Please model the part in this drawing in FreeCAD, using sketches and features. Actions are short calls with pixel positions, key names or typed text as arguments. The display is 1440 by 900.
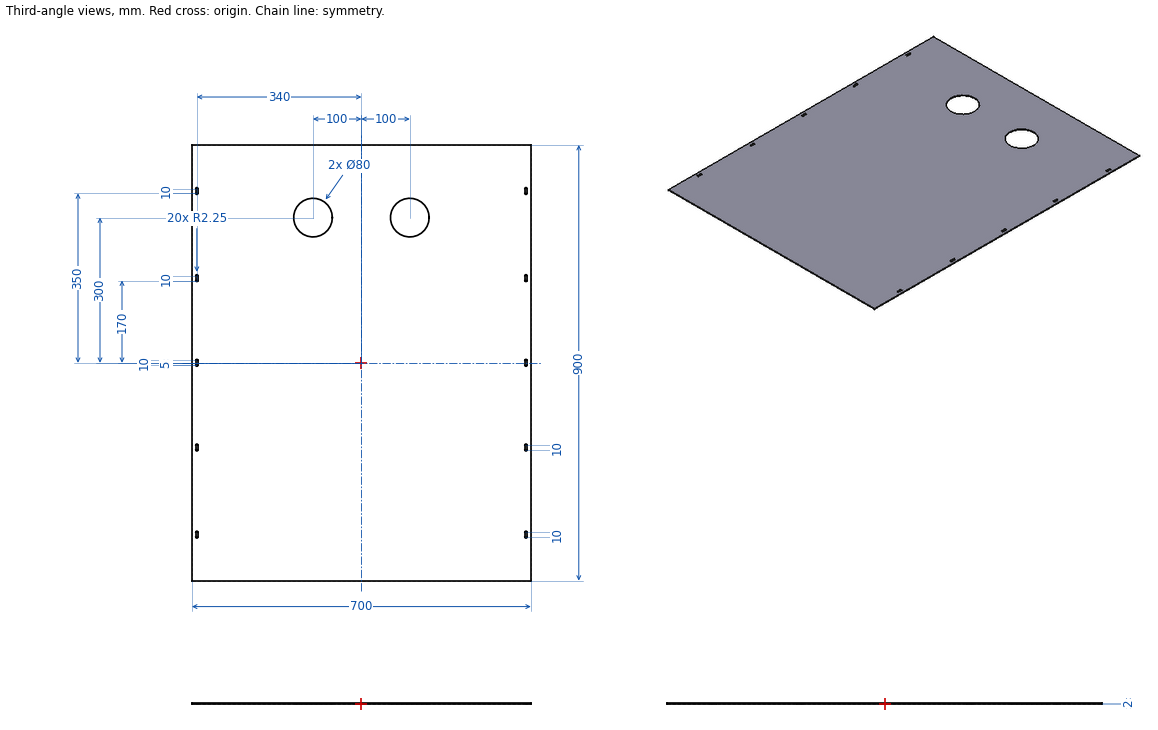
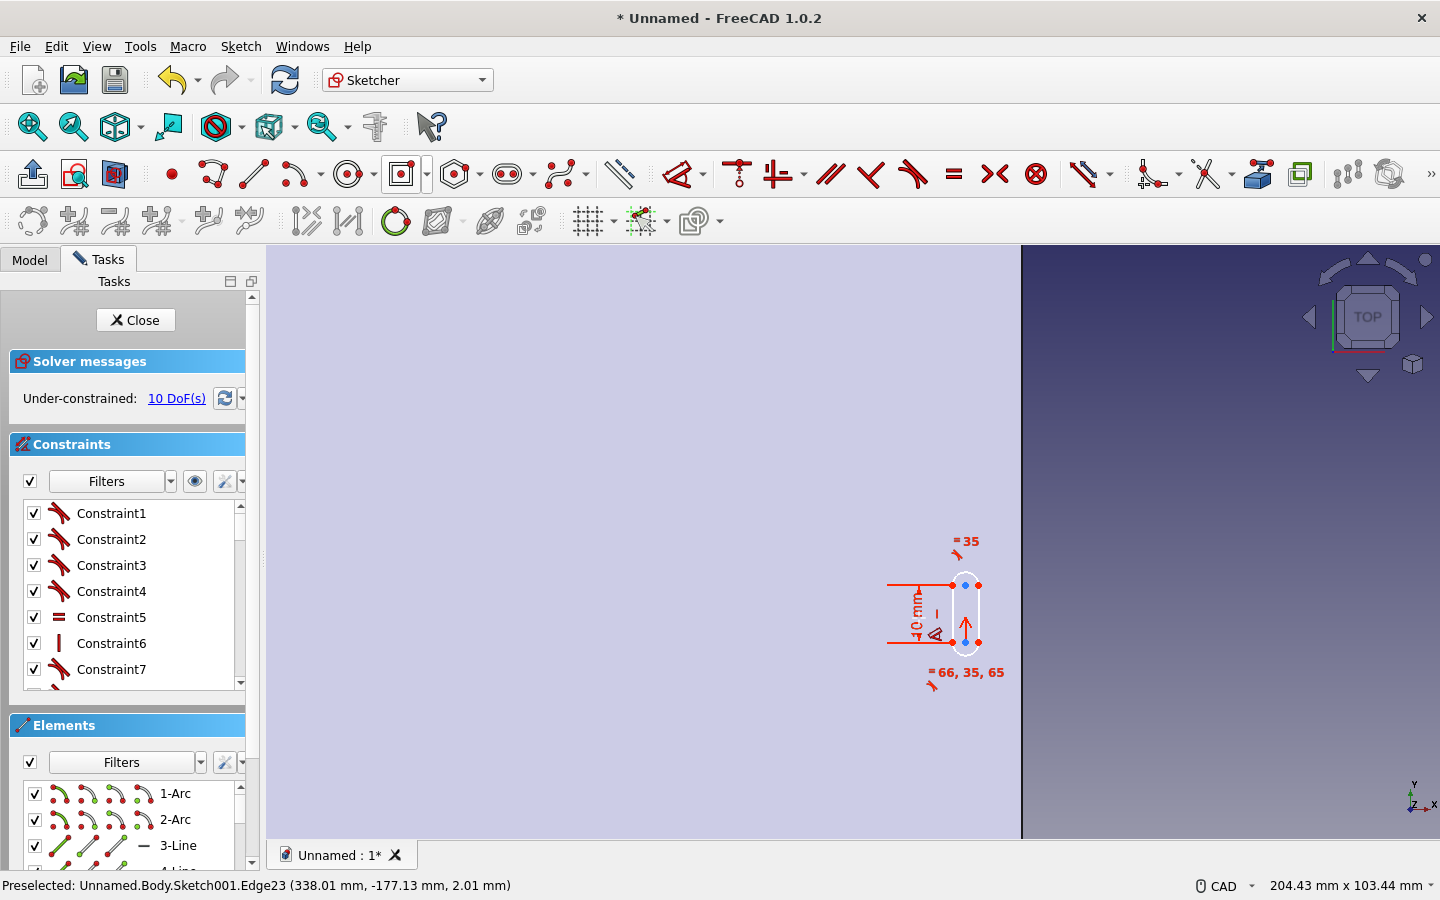
scroll(961, 635, down, 12)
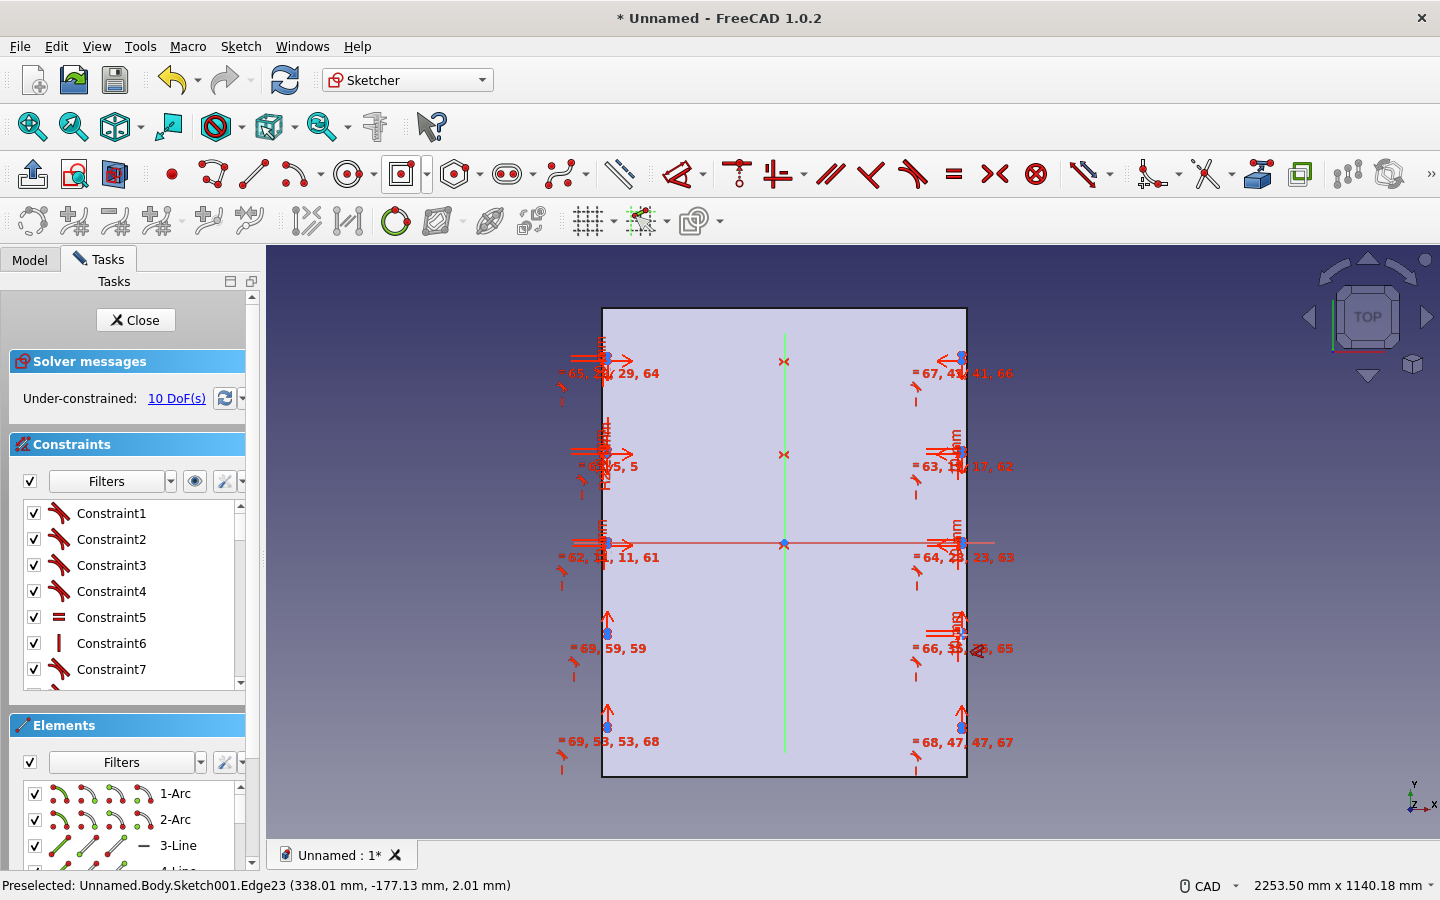
scroll(961, 359, up, 11)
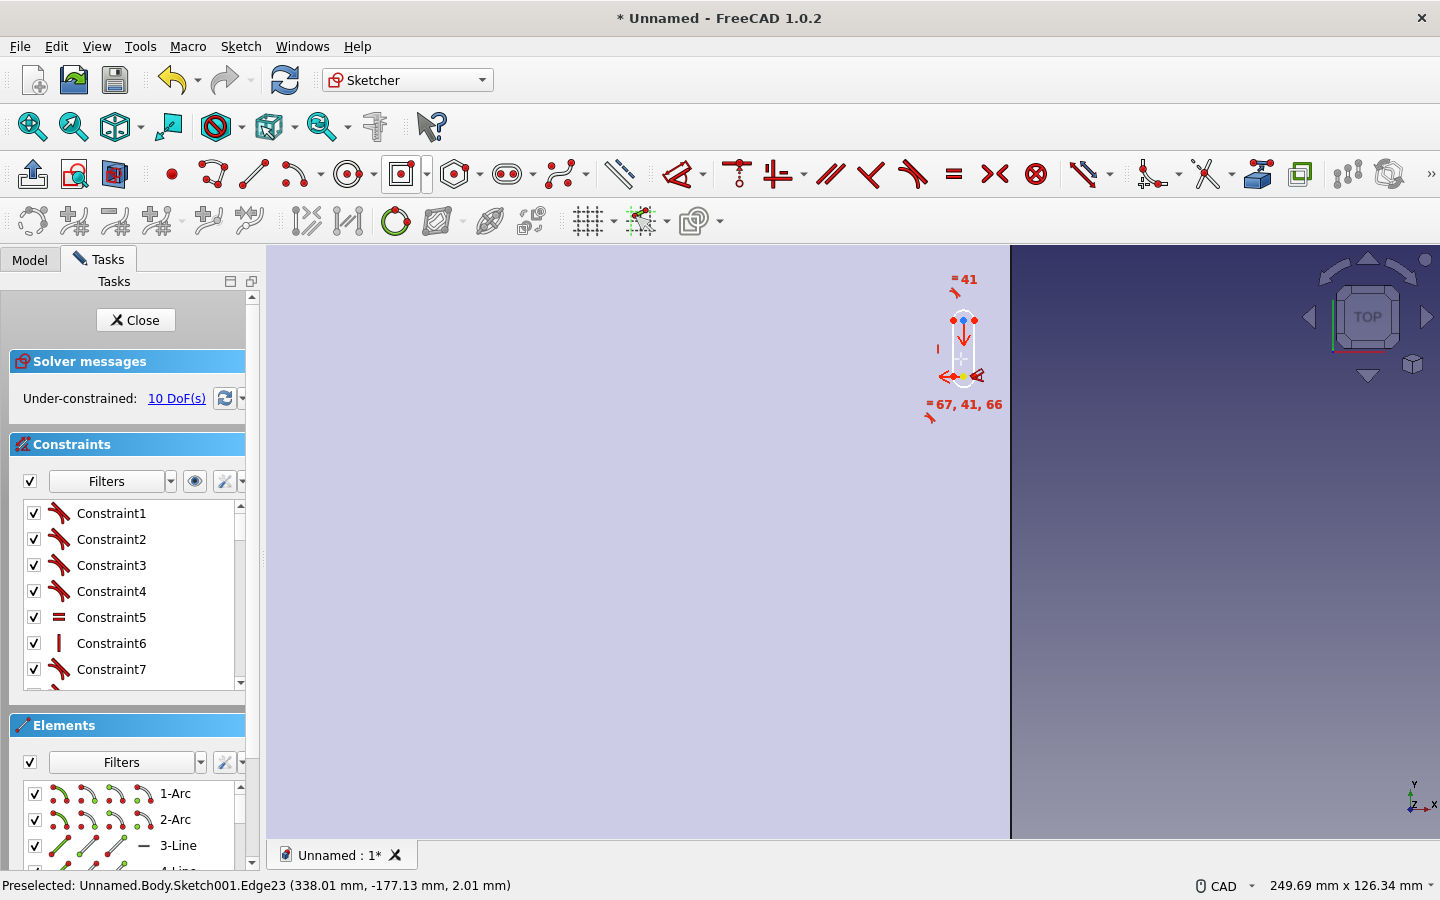
click(953, 360)
click(919, 349)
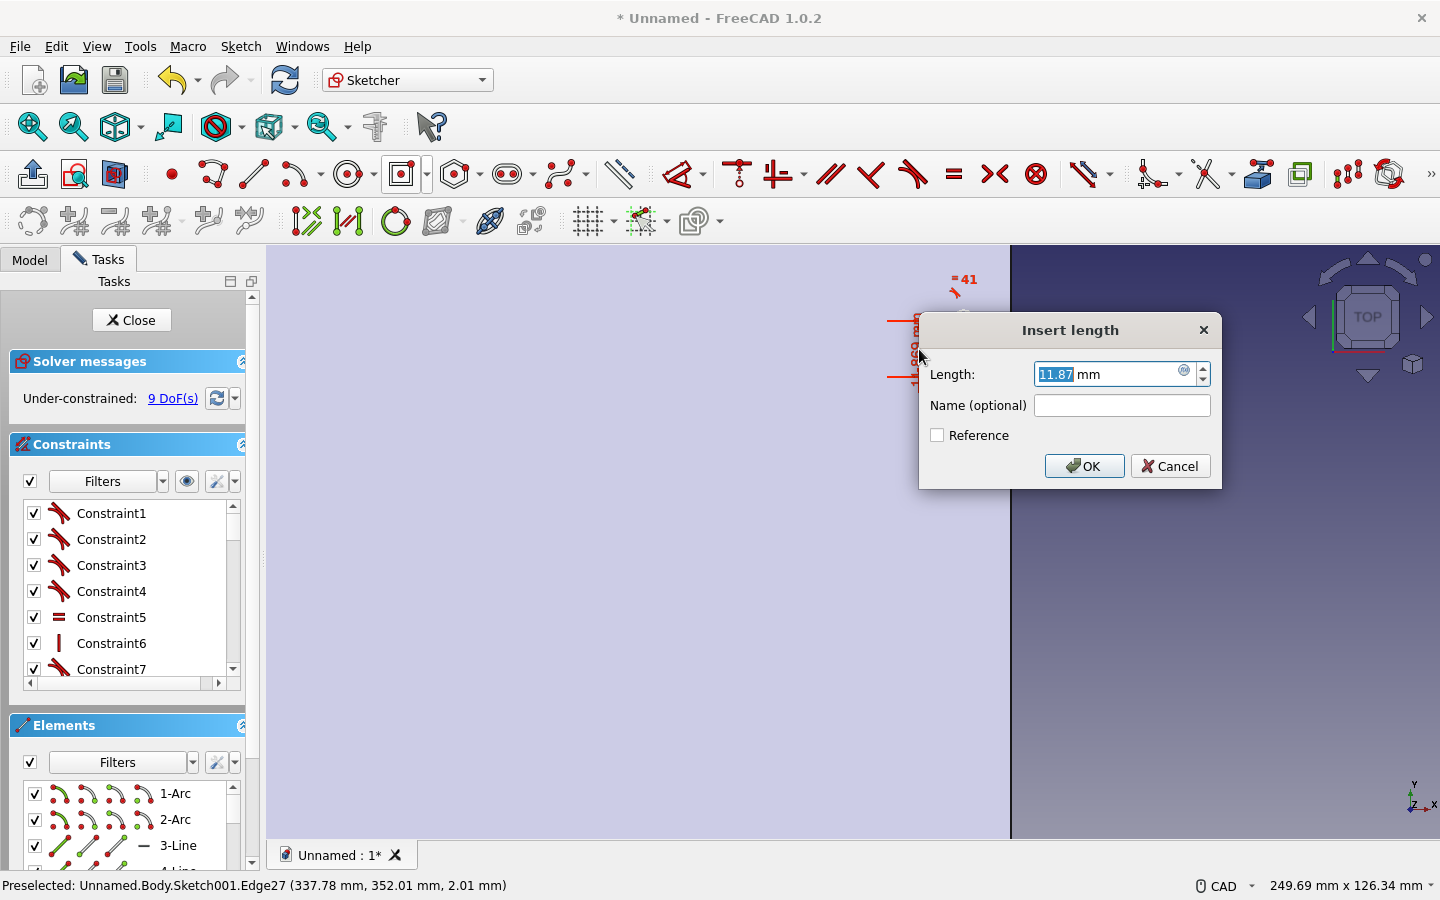
text(10)
key(Return)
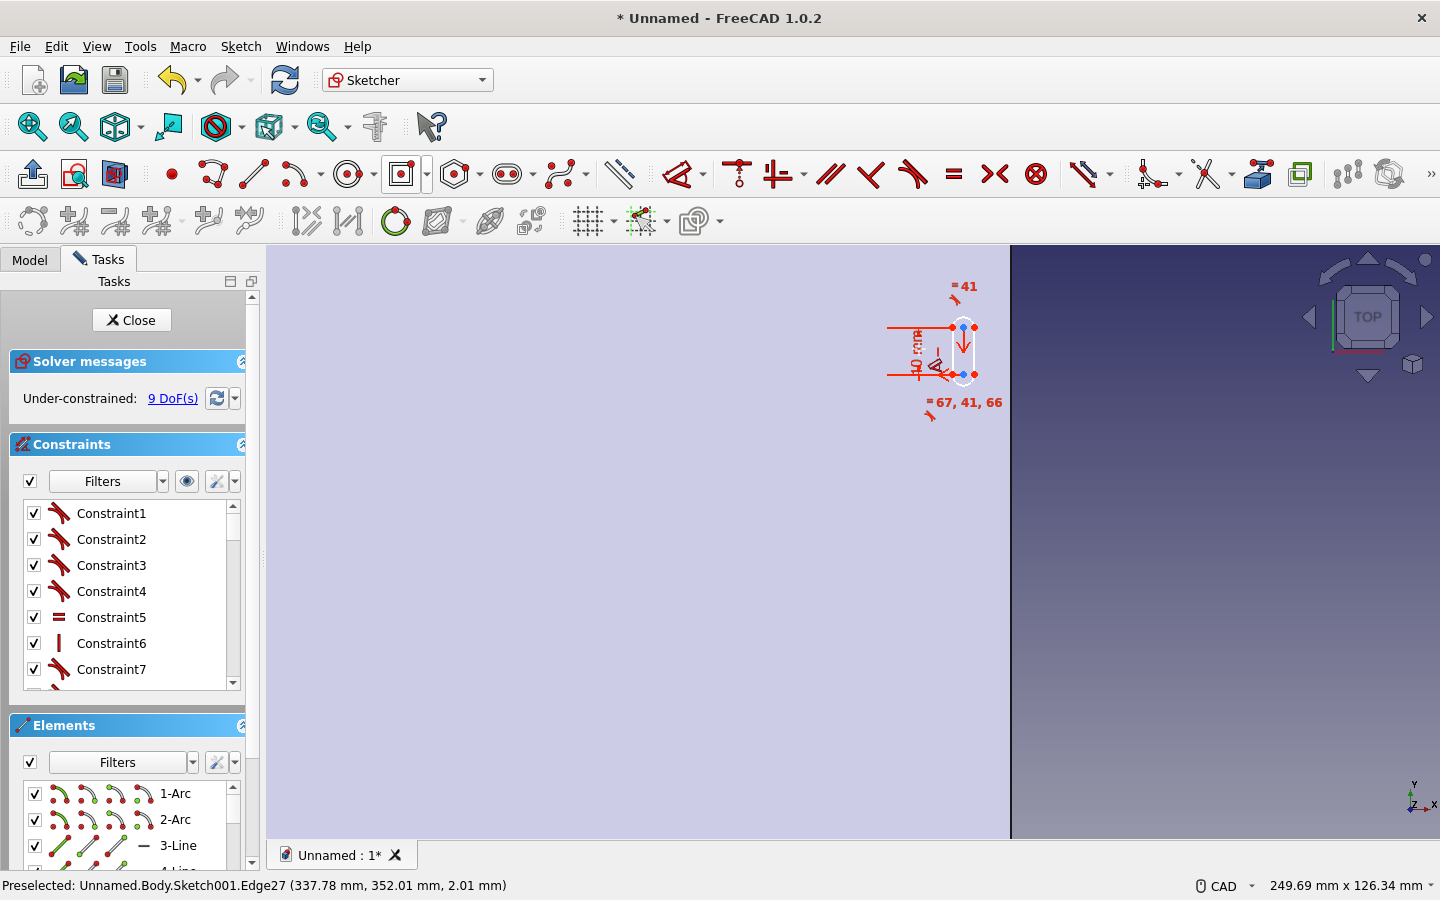
scroll(961, 358, down, 11)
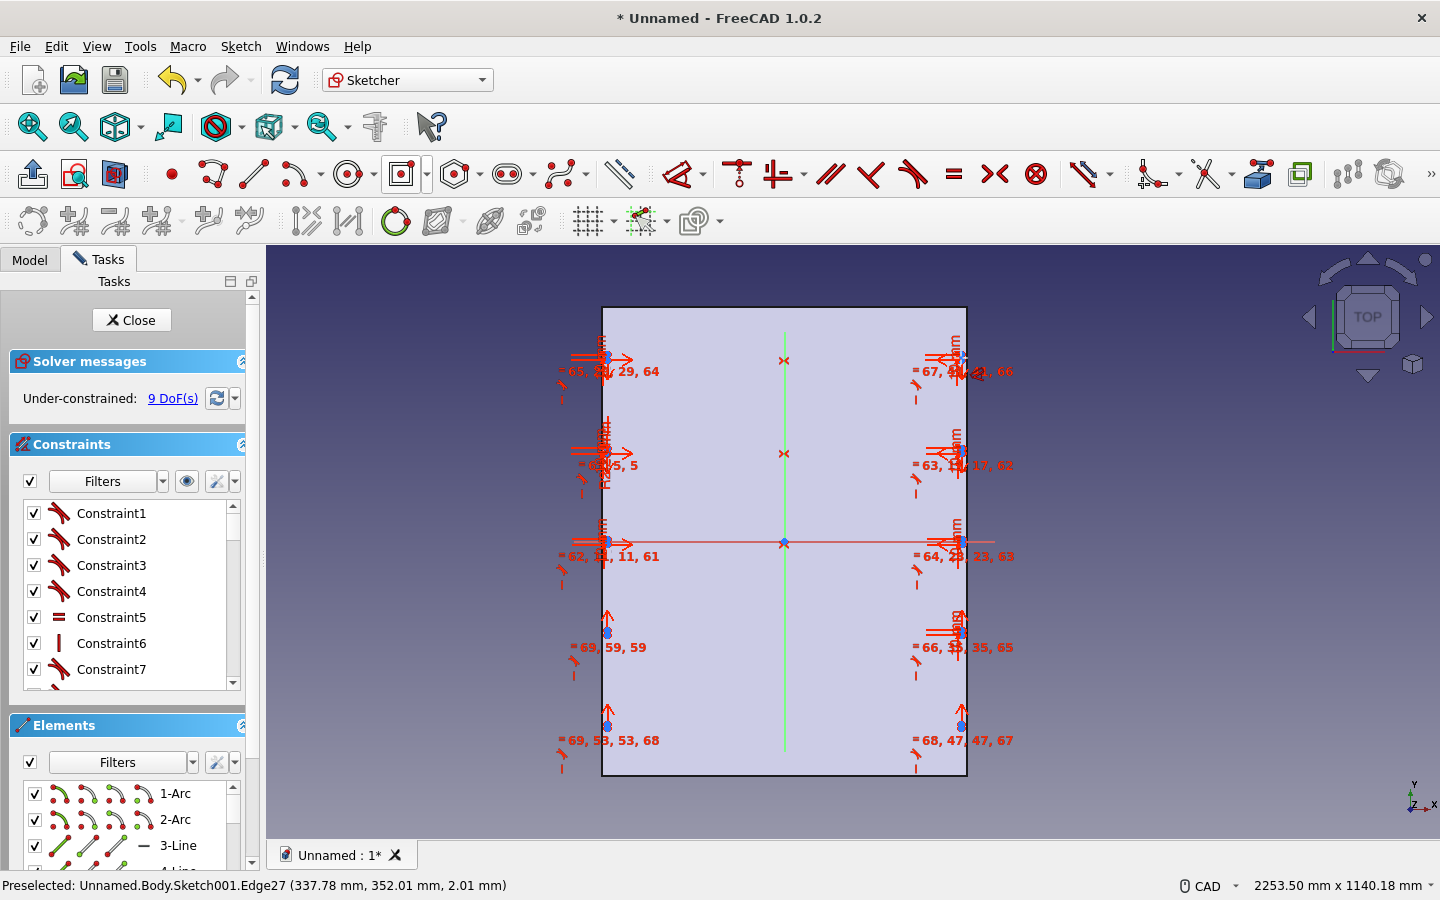
scroll(961, 728, up, 12)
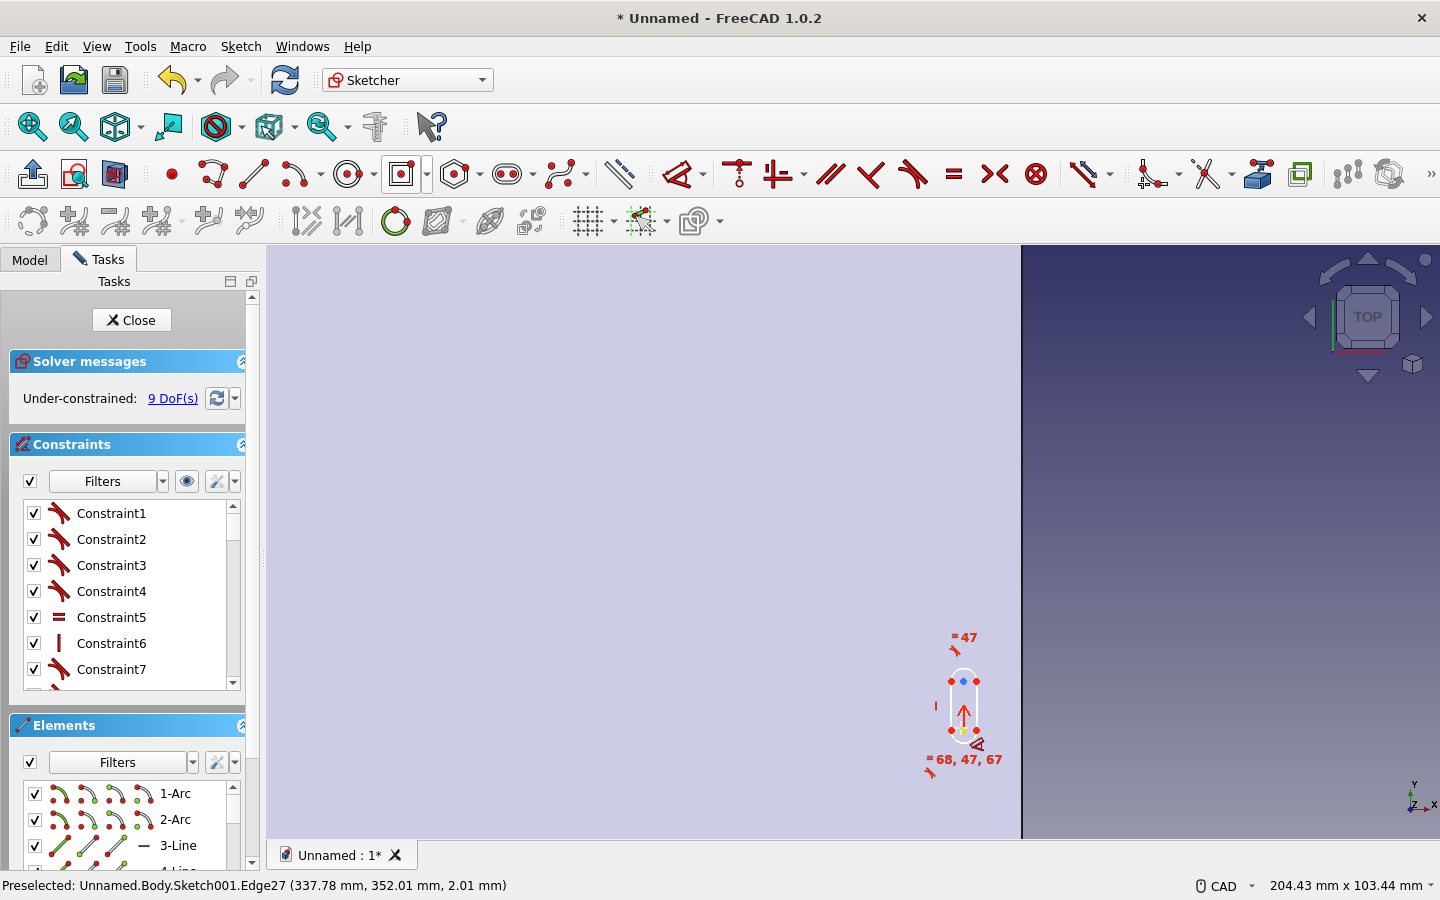
click(951, 716)
click(917, 706)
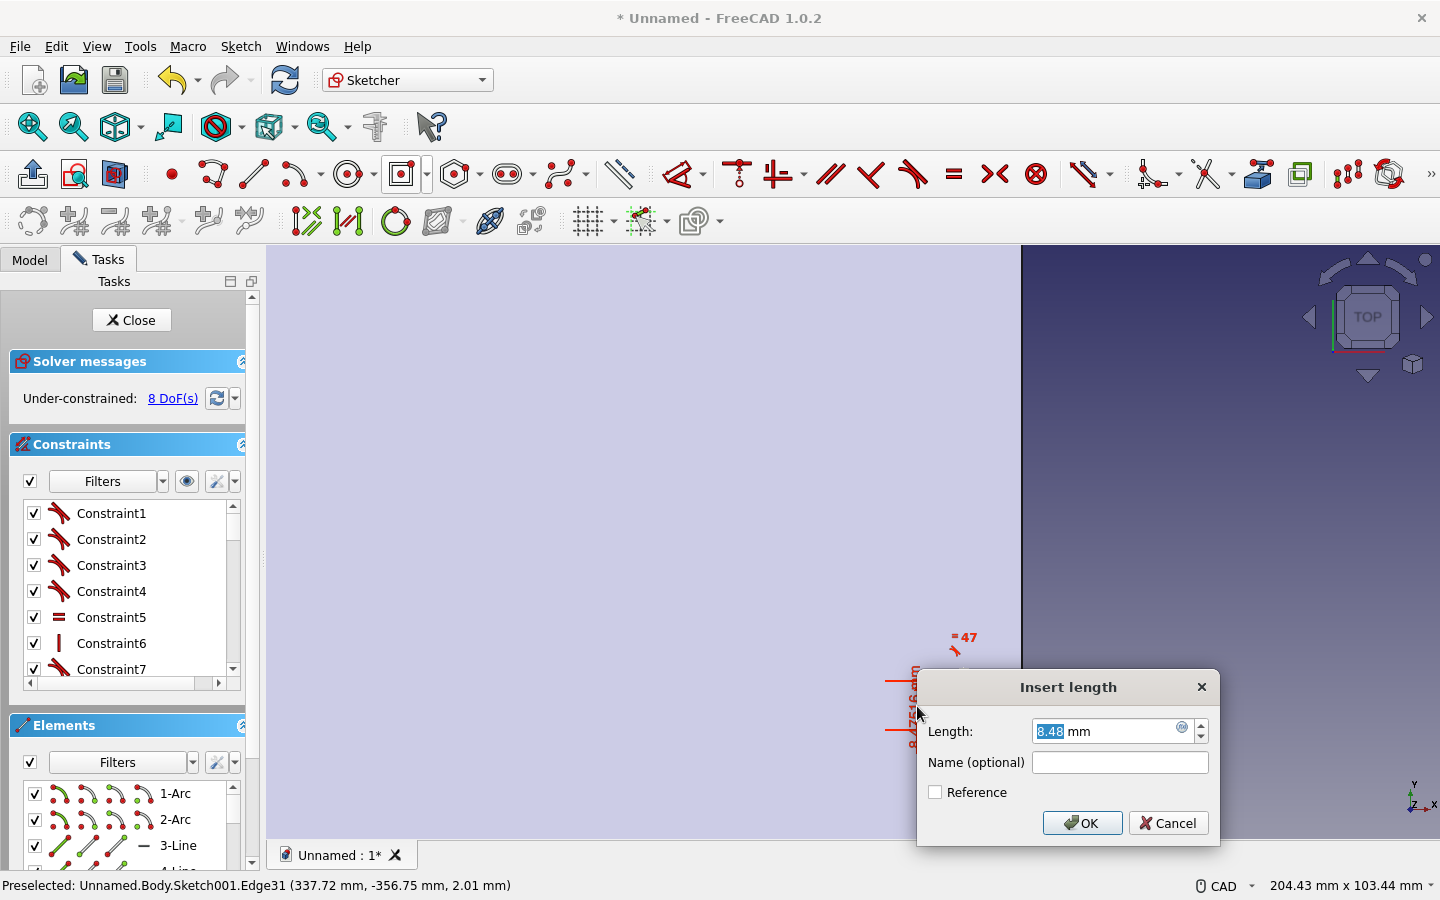
text(10)
key(Return)